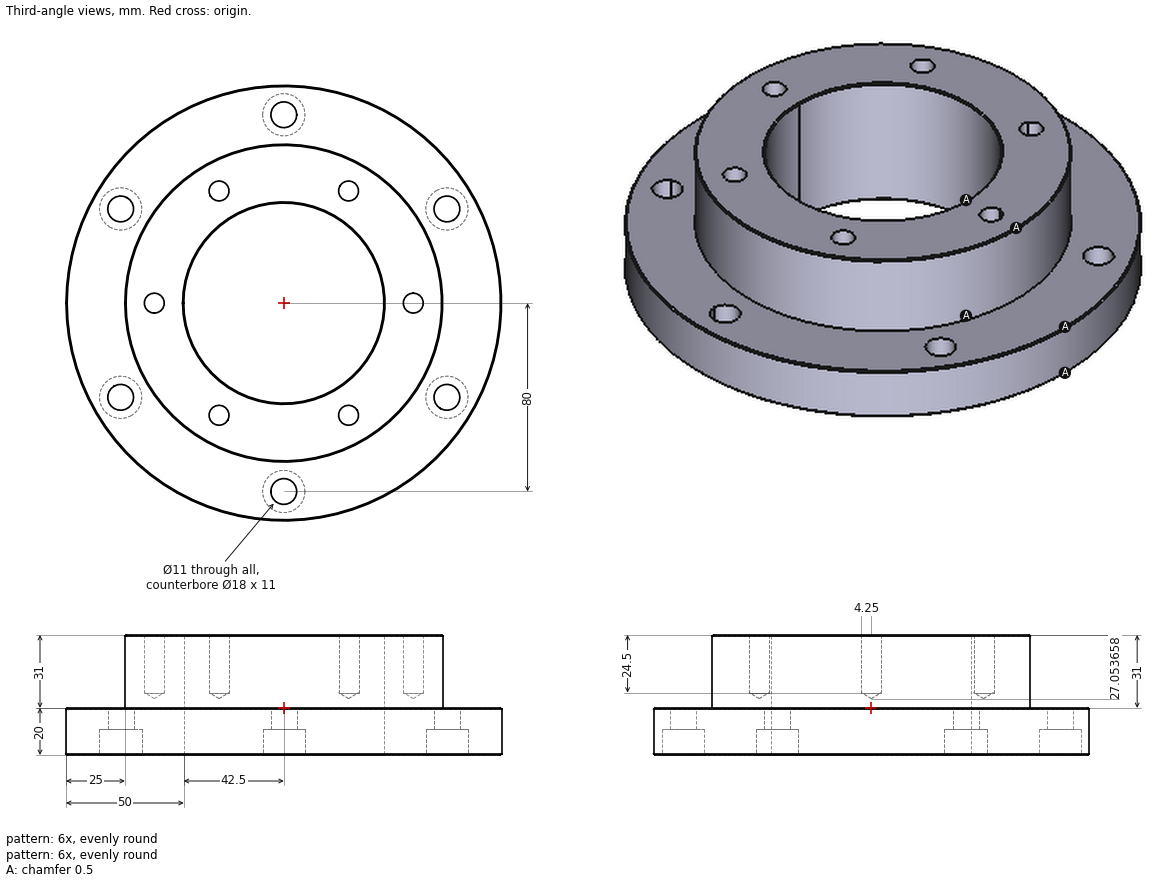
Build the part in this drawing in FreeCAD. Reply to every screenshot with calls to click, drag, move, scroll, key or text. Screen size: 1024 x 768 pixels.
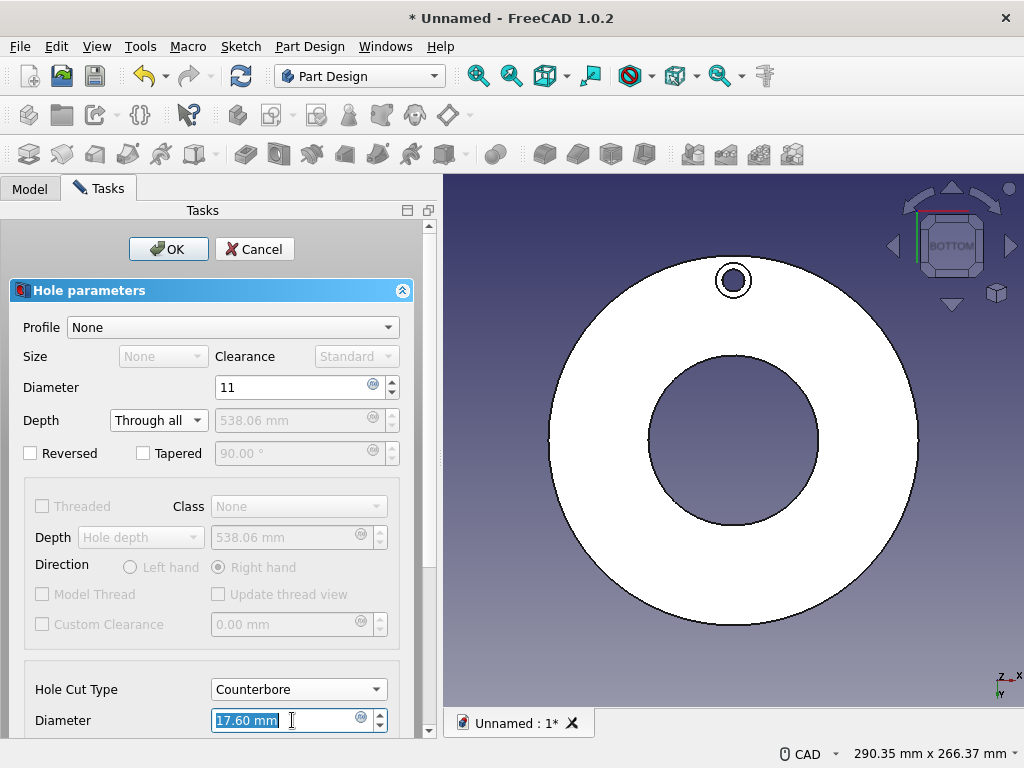
text(18)
key(Tab)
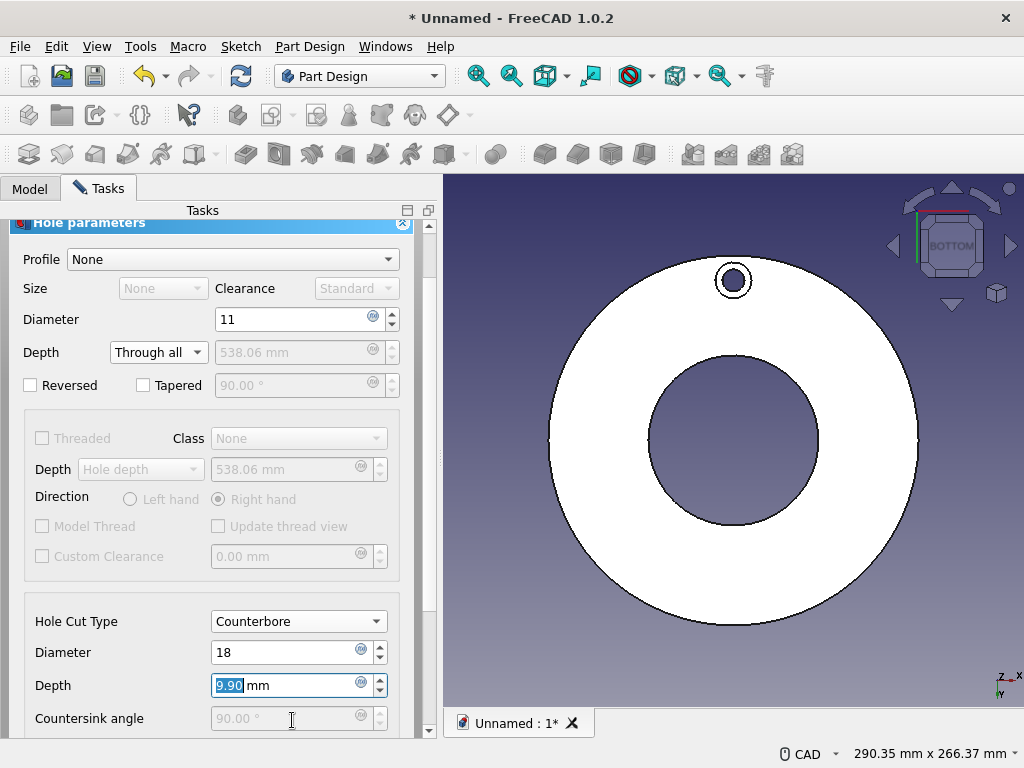
text(11)
key(Tab)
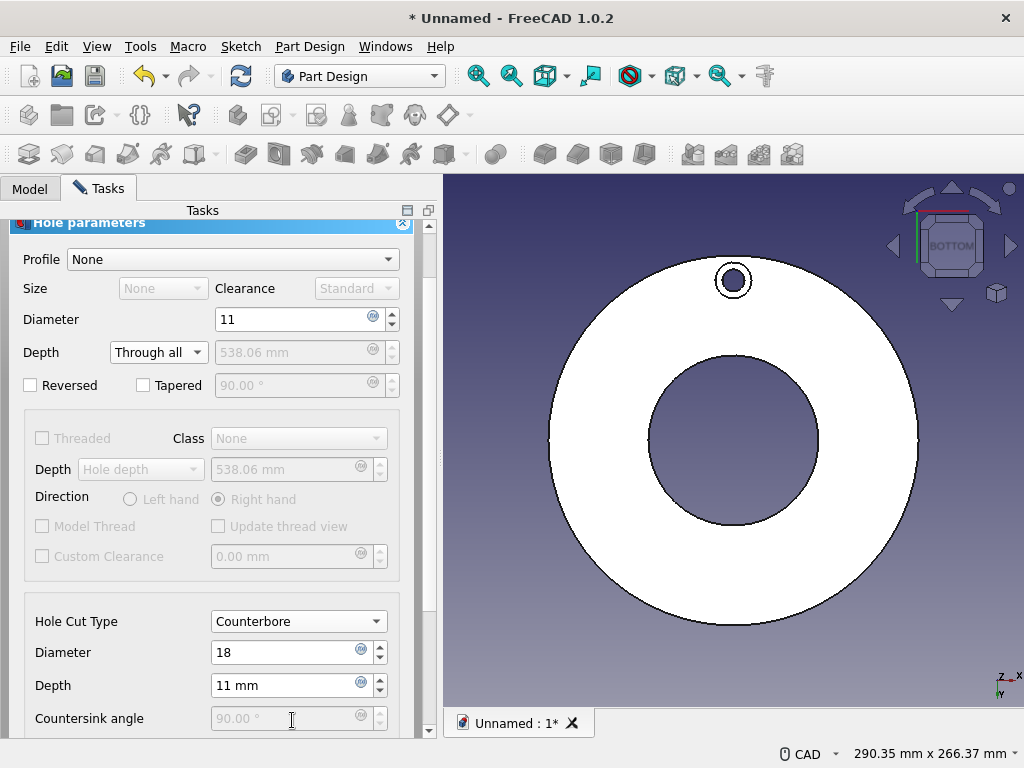
scroll(429, 479, up, 2)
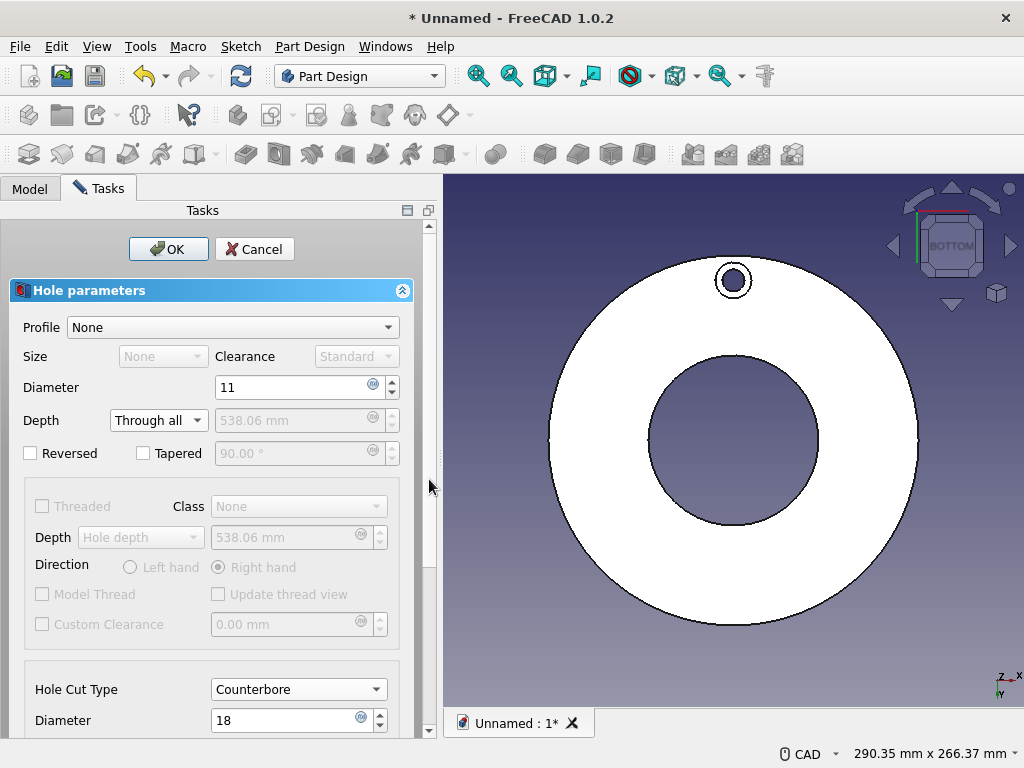
click(169, 249)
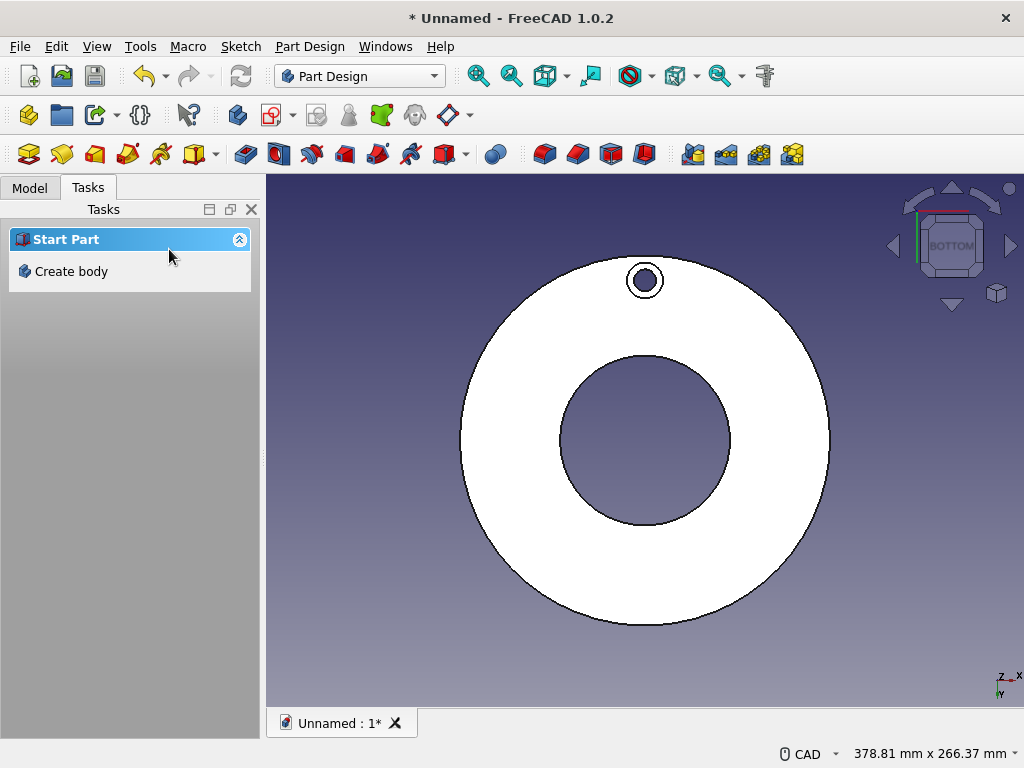
click(30, 188)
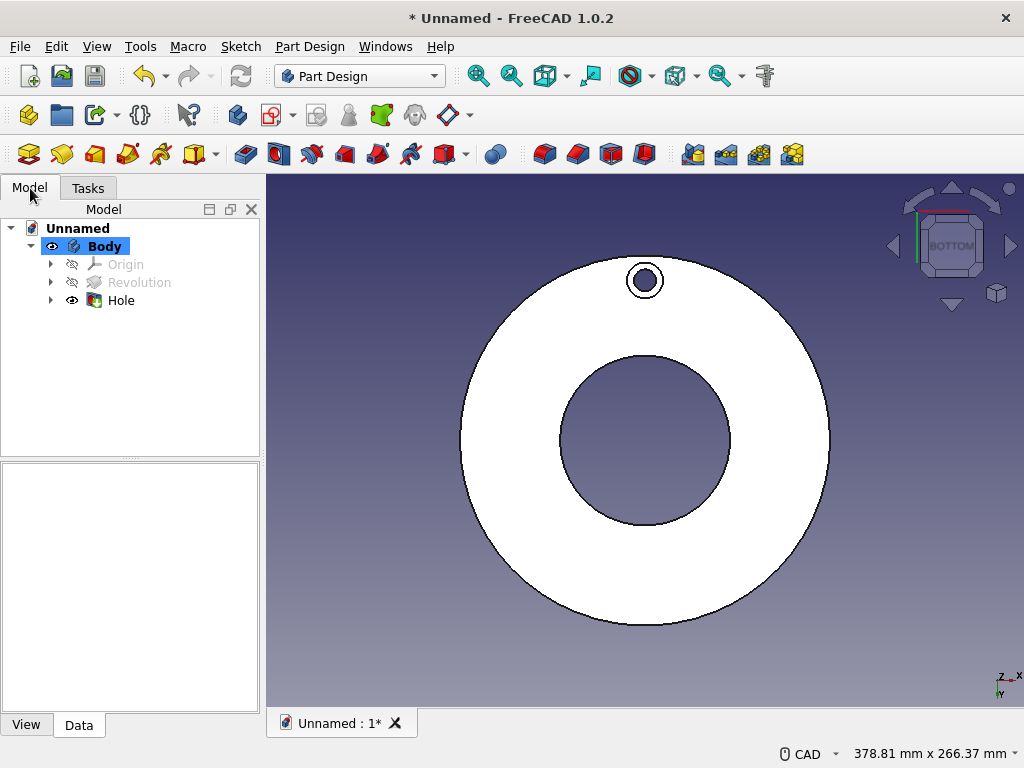
click(117, 300)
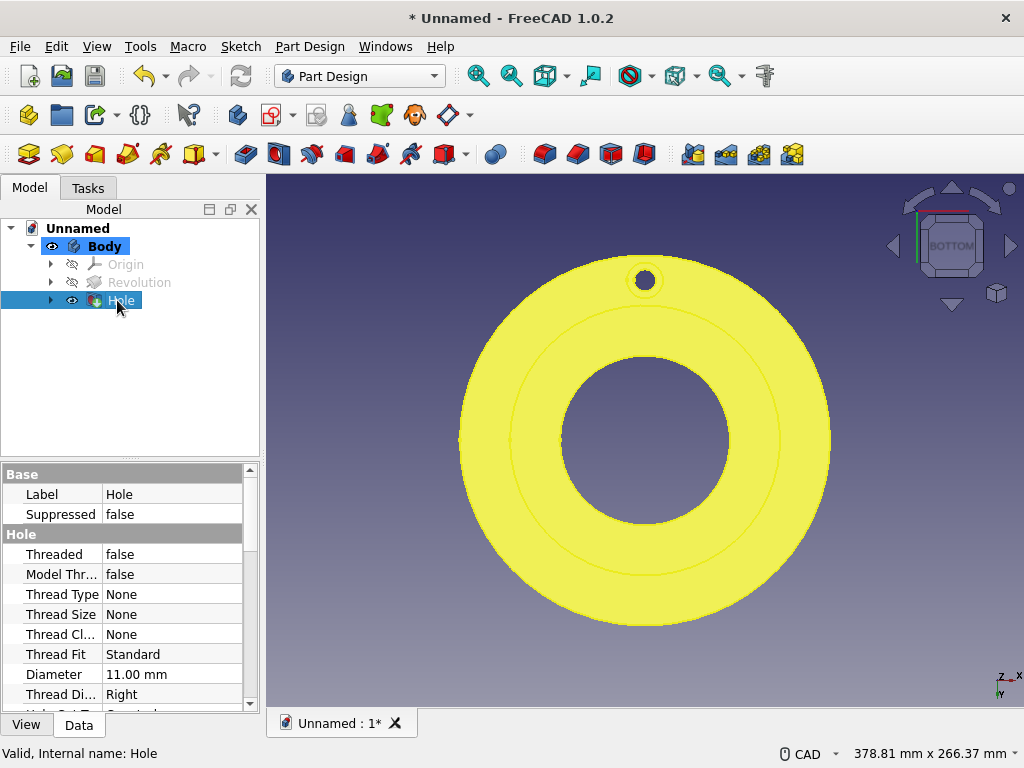
click(759, 154)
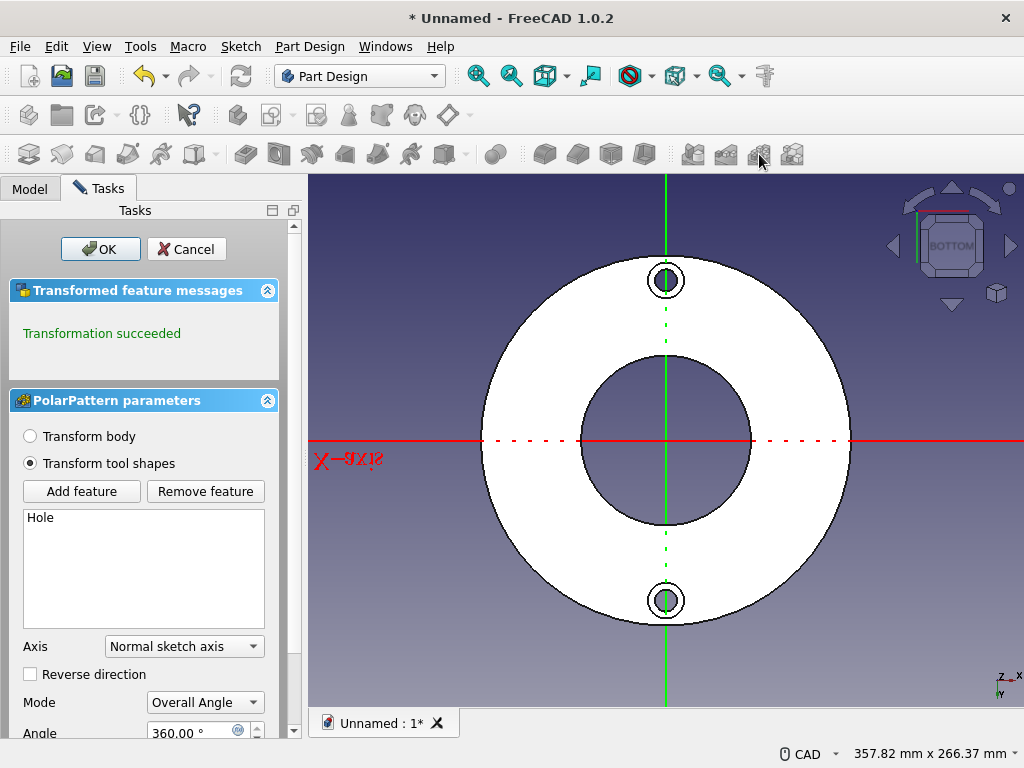
click(185, 646)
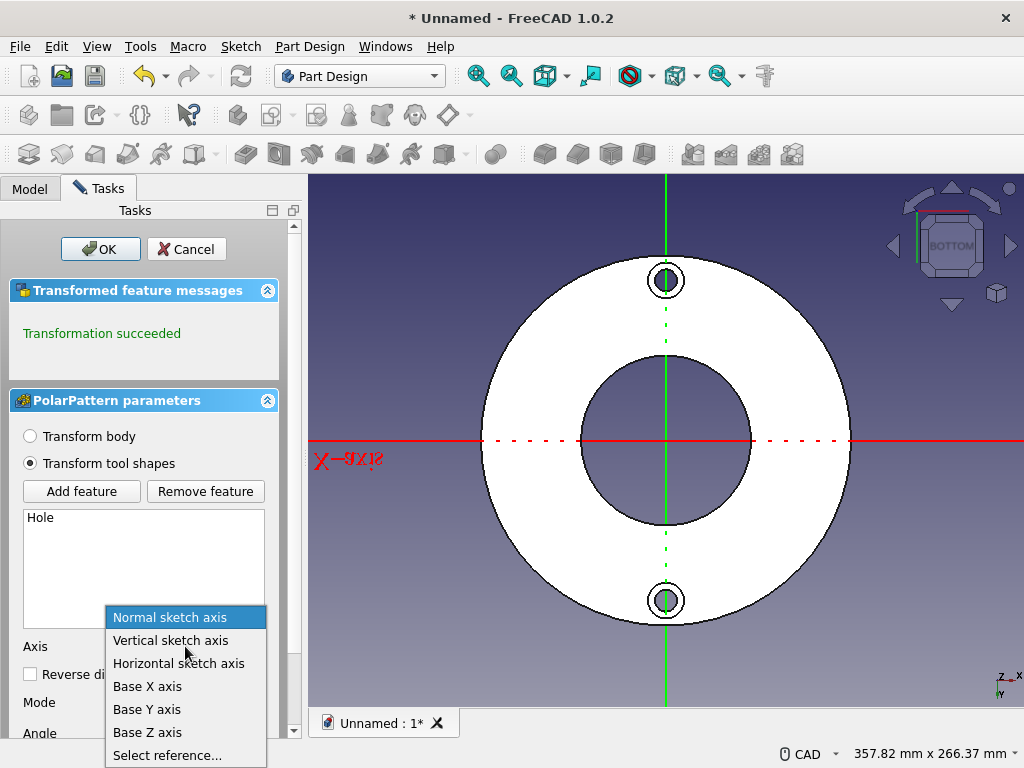
click(184, 732)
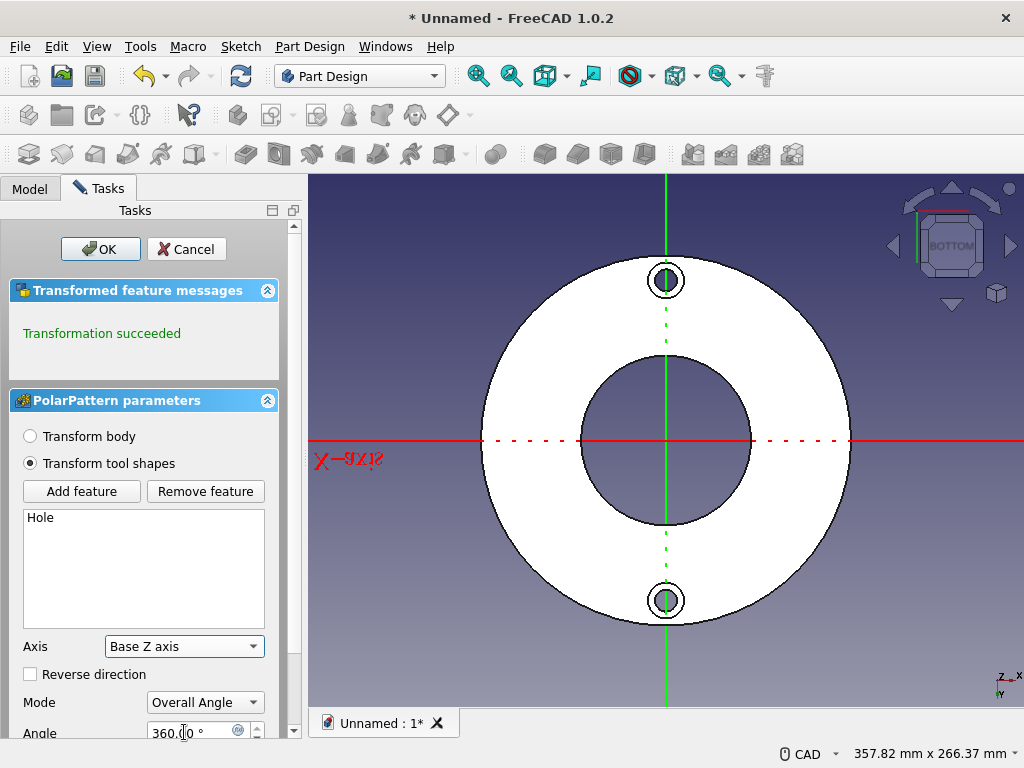
scroll(294, 479, down, 2)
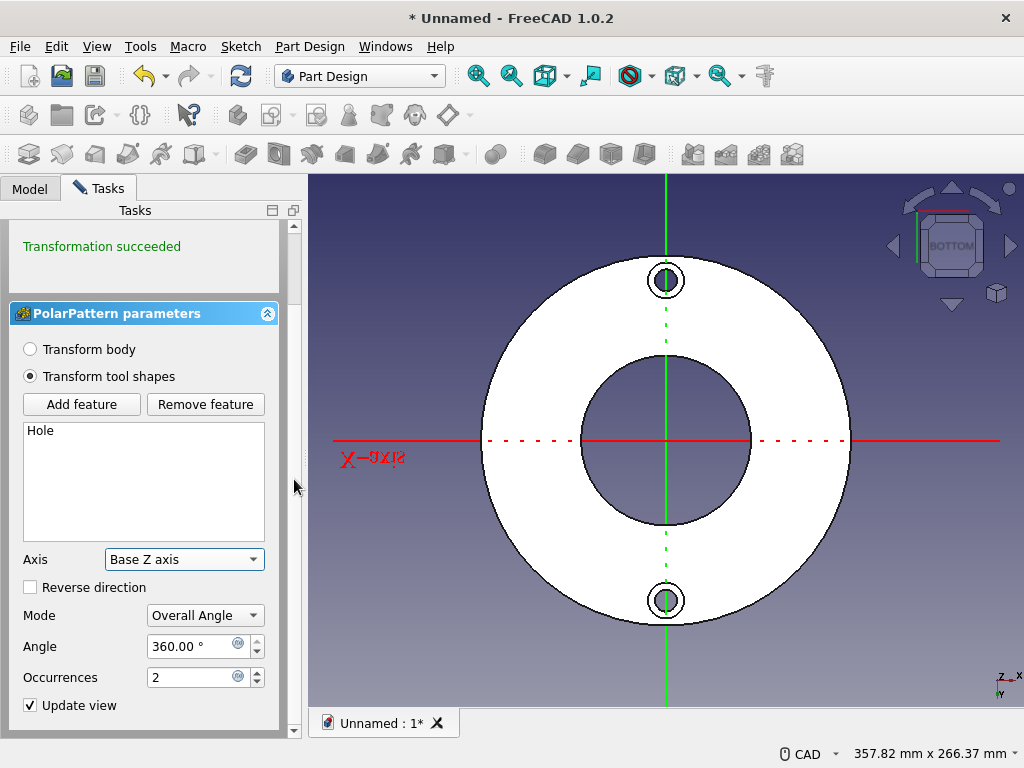
triple_click(199, 678)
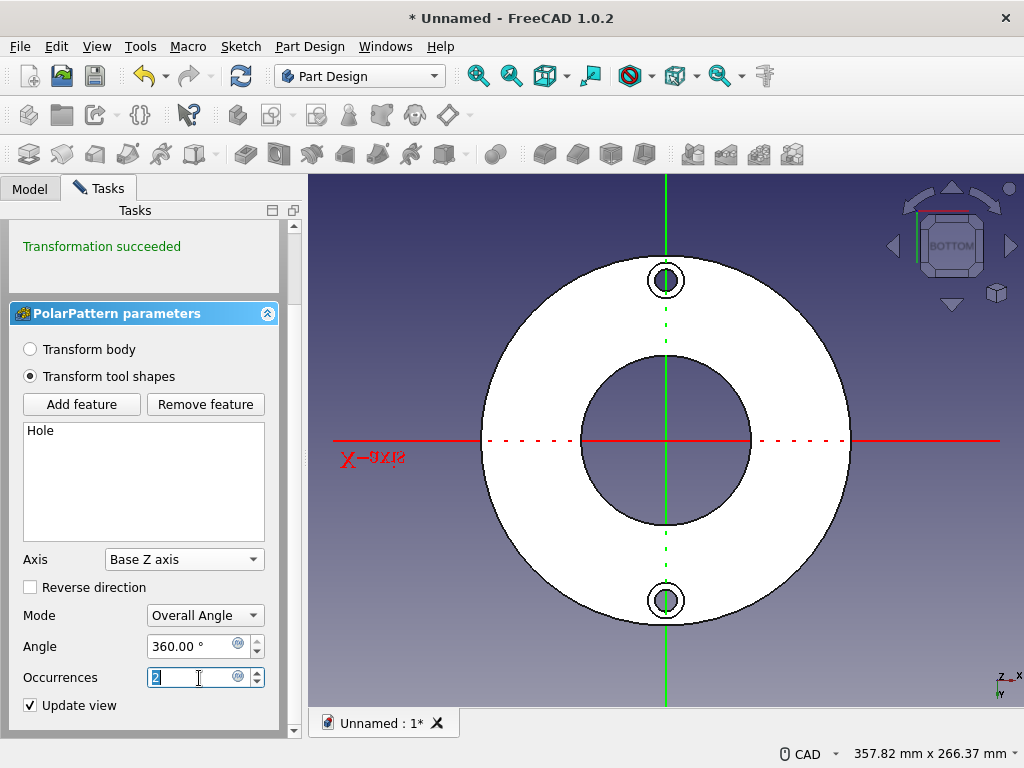
text(6)
key(Tab)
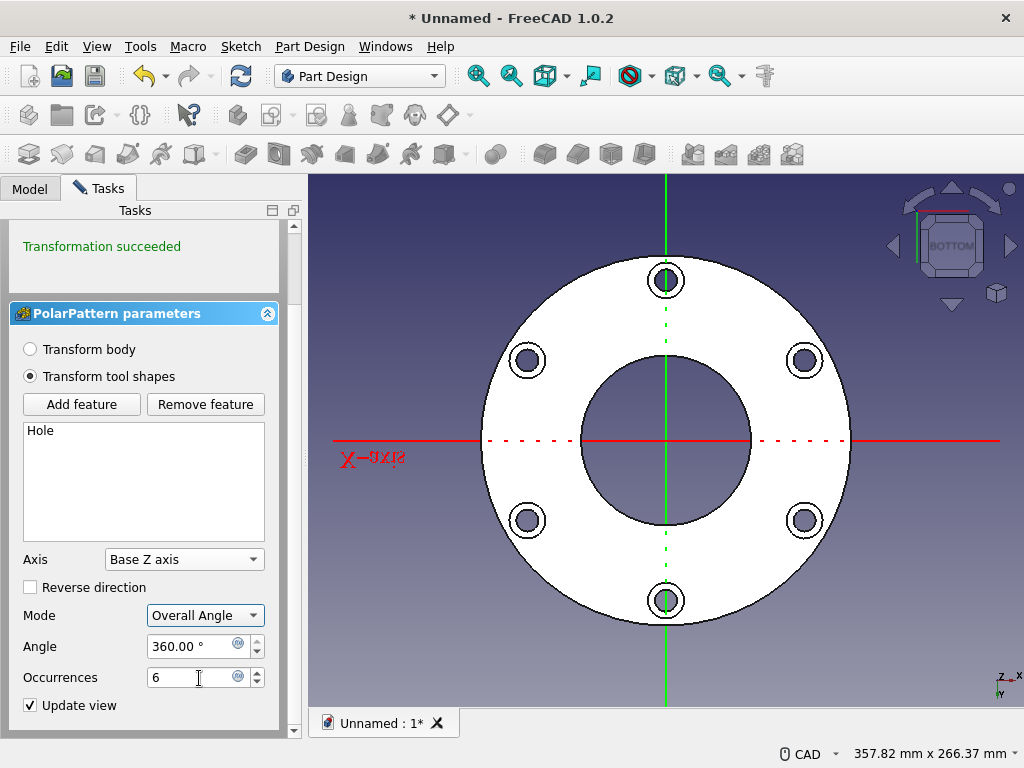
scroll(294, 479, up, 3)